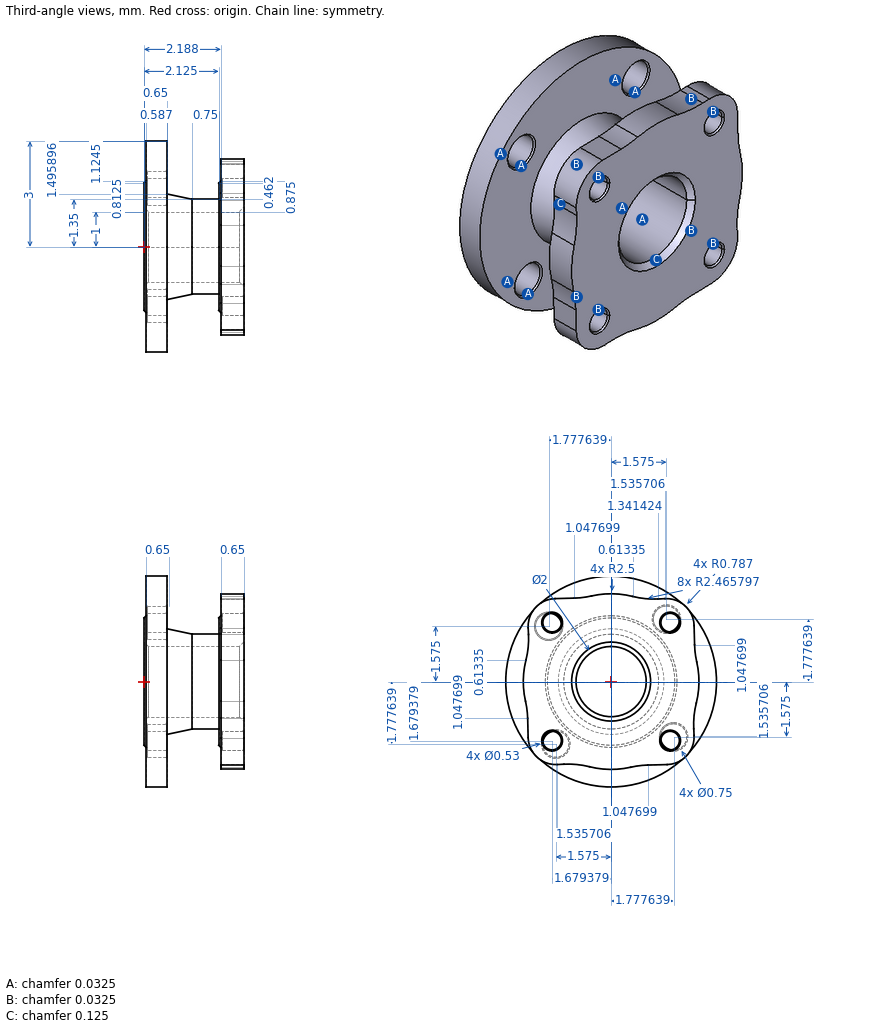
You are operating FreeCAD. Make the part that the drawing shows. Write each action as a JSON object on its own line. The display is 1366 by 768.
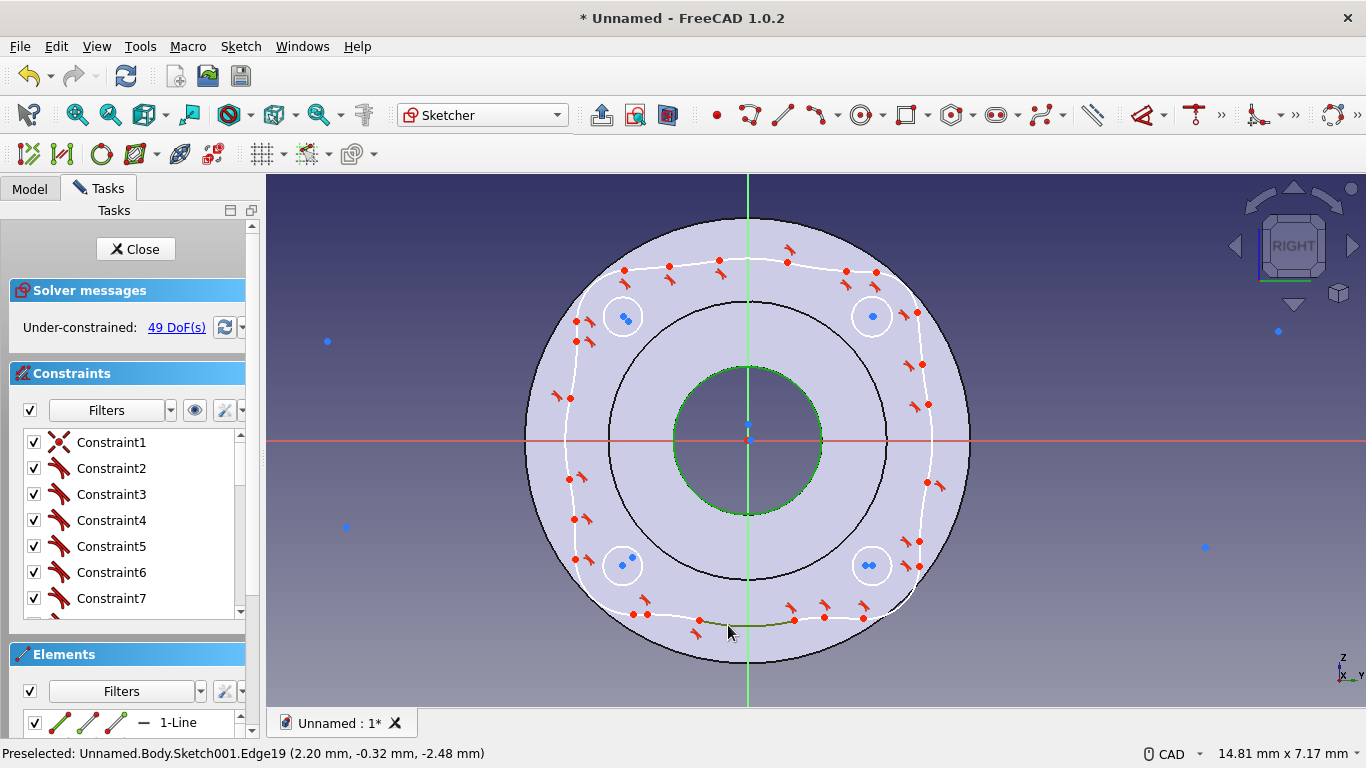
{"action": "left_click", "coordinate": [1194, 116]}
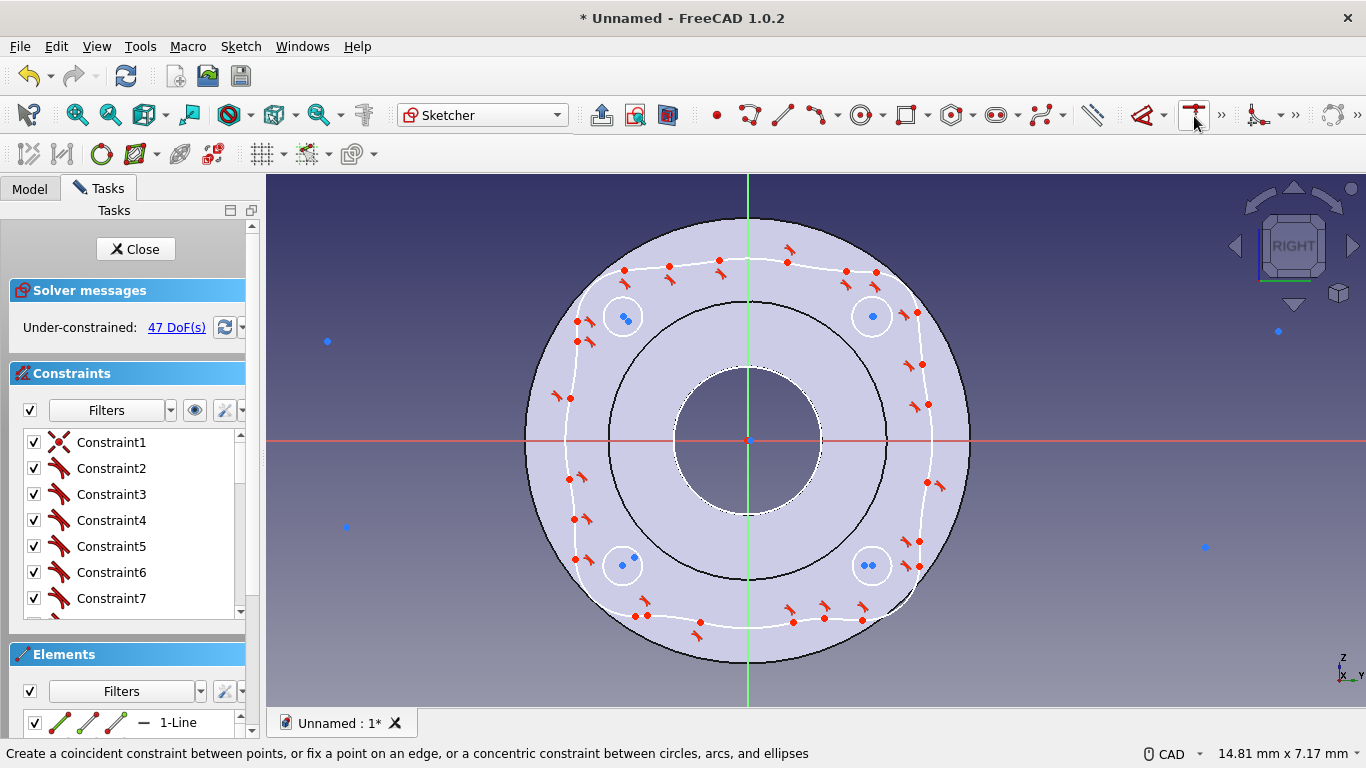
{"action": "left_click", "coordinate": [800, 388]}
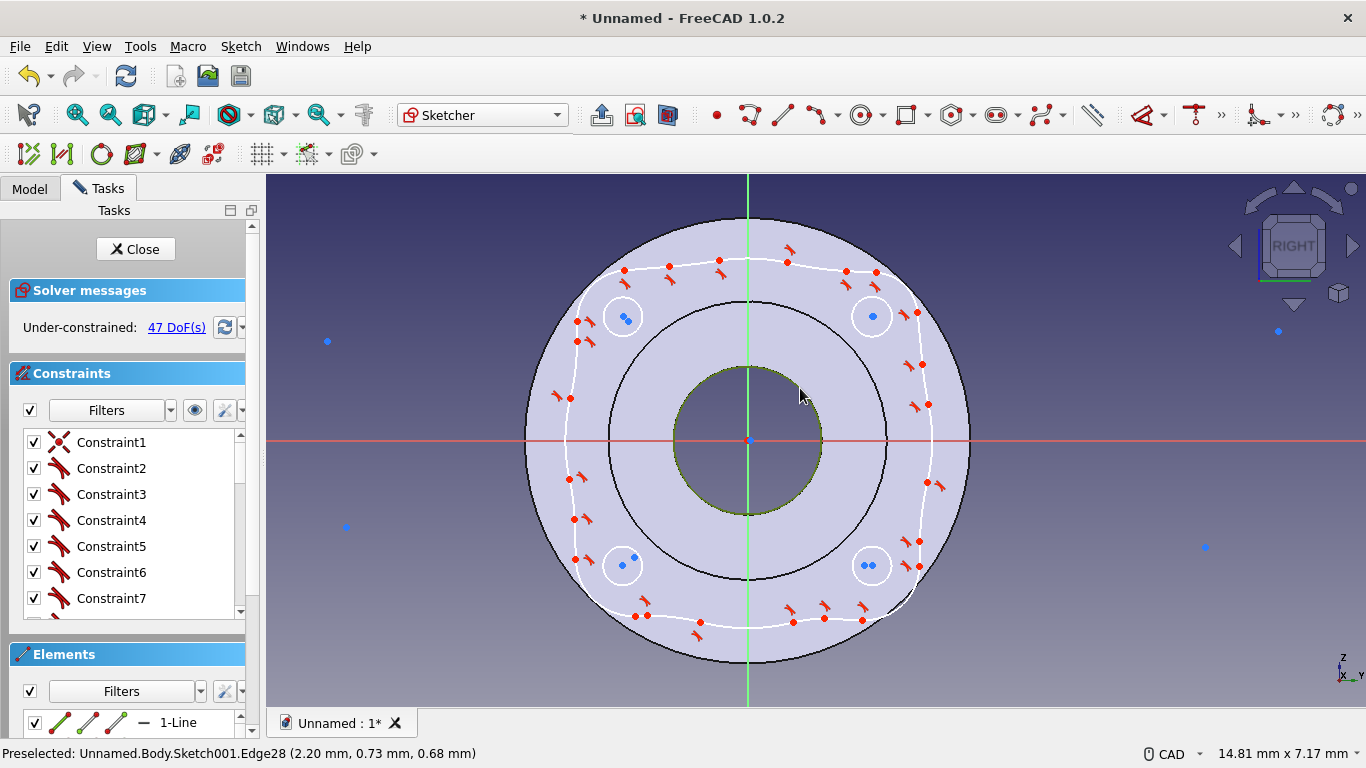
{"action": "left_click", "coordinate": [931, 459]}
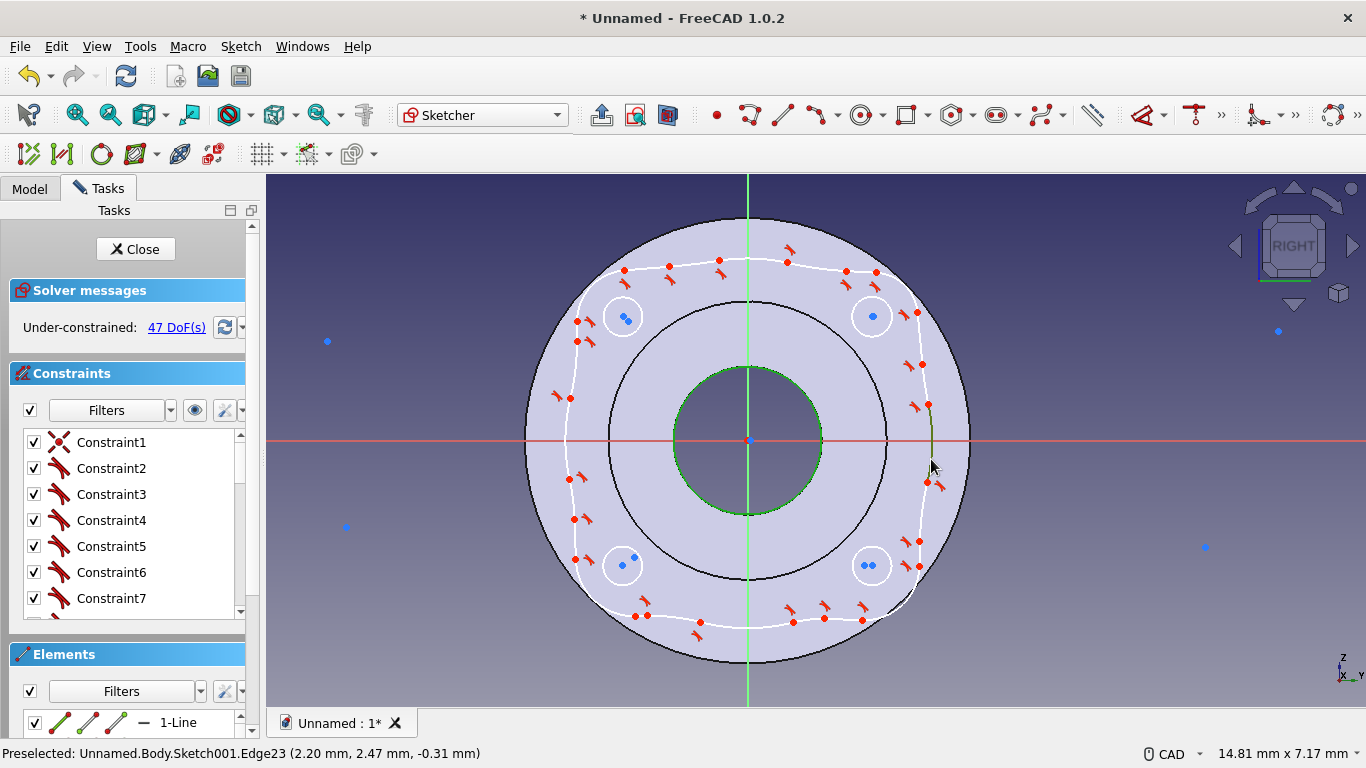
{"action": "left_click", "coordinate": [1194, 116]}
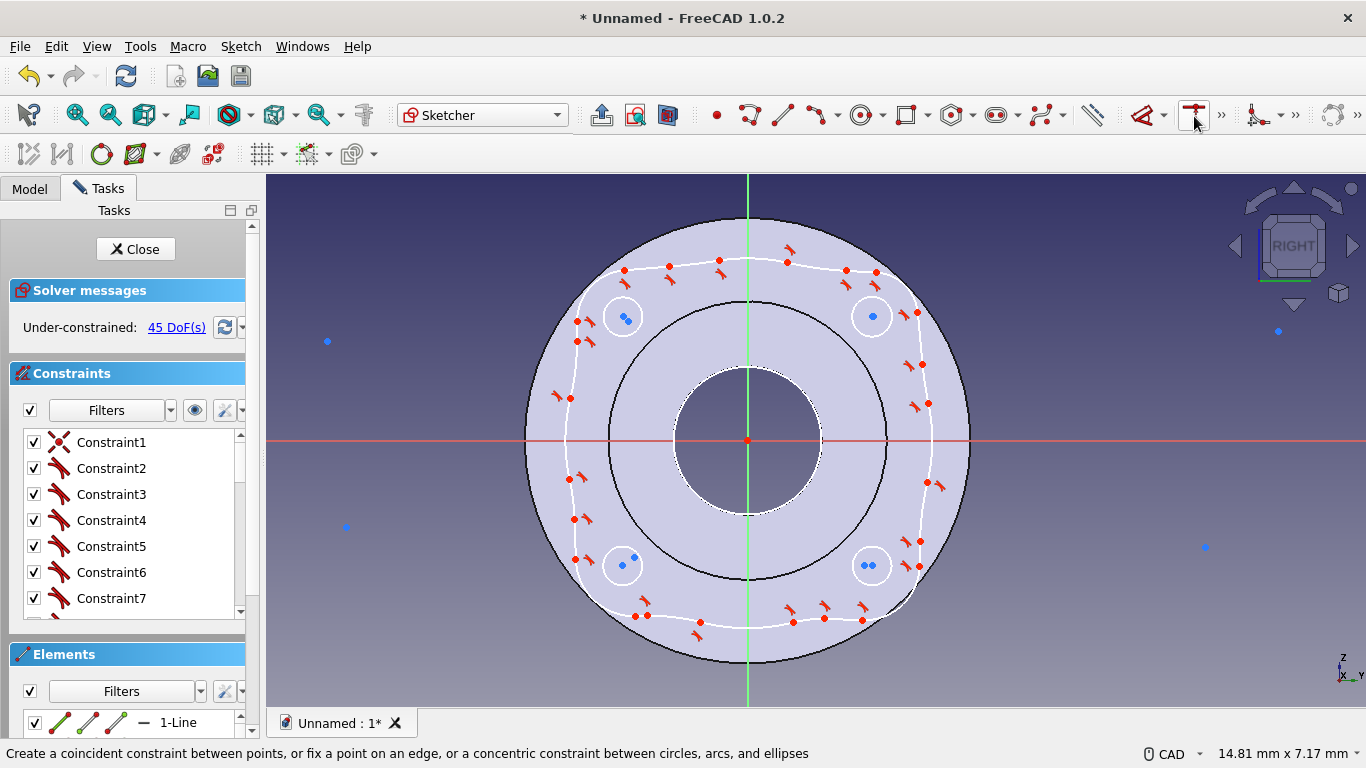
{"action": "left_click", "coordinate": [805, 266]}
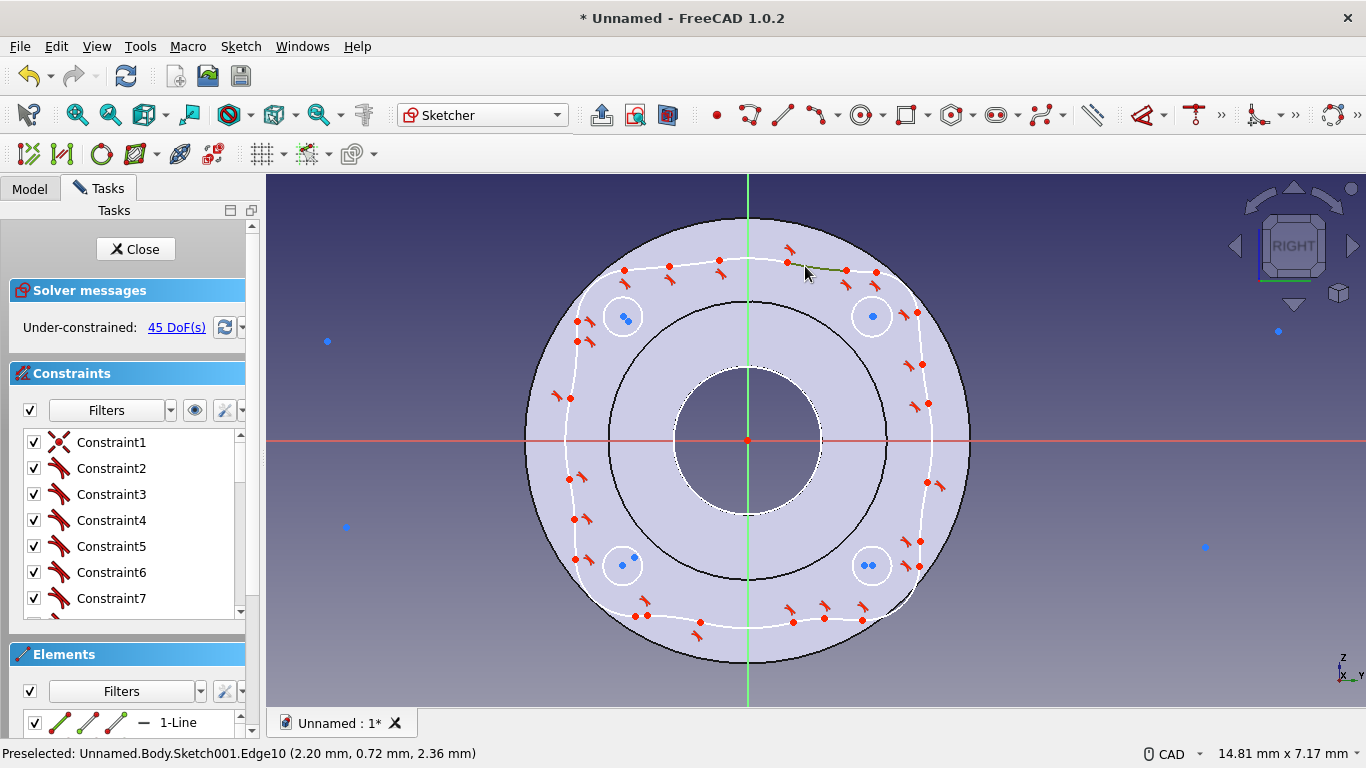
{"action": "left_click", "coordinate": [684, 265]}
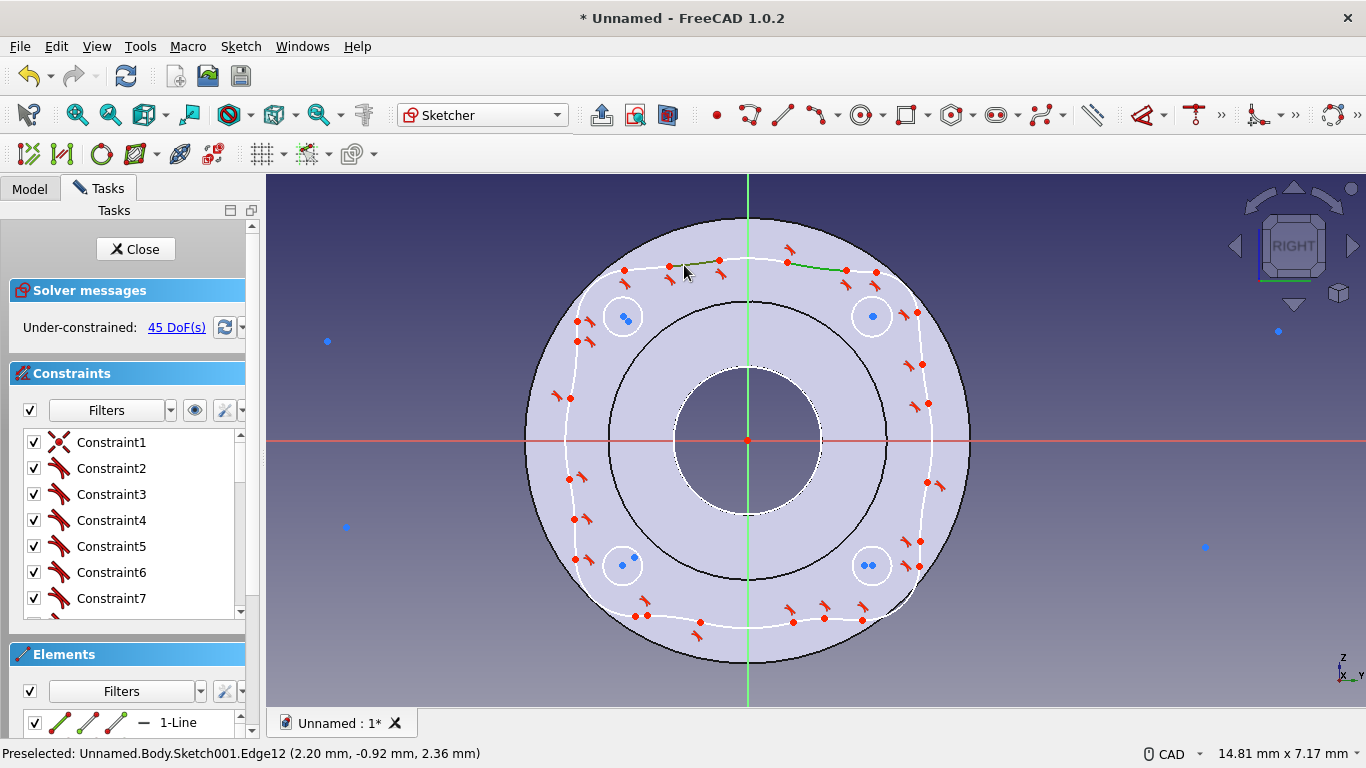
{"action": "left_click", "coordinate": [574, 382]}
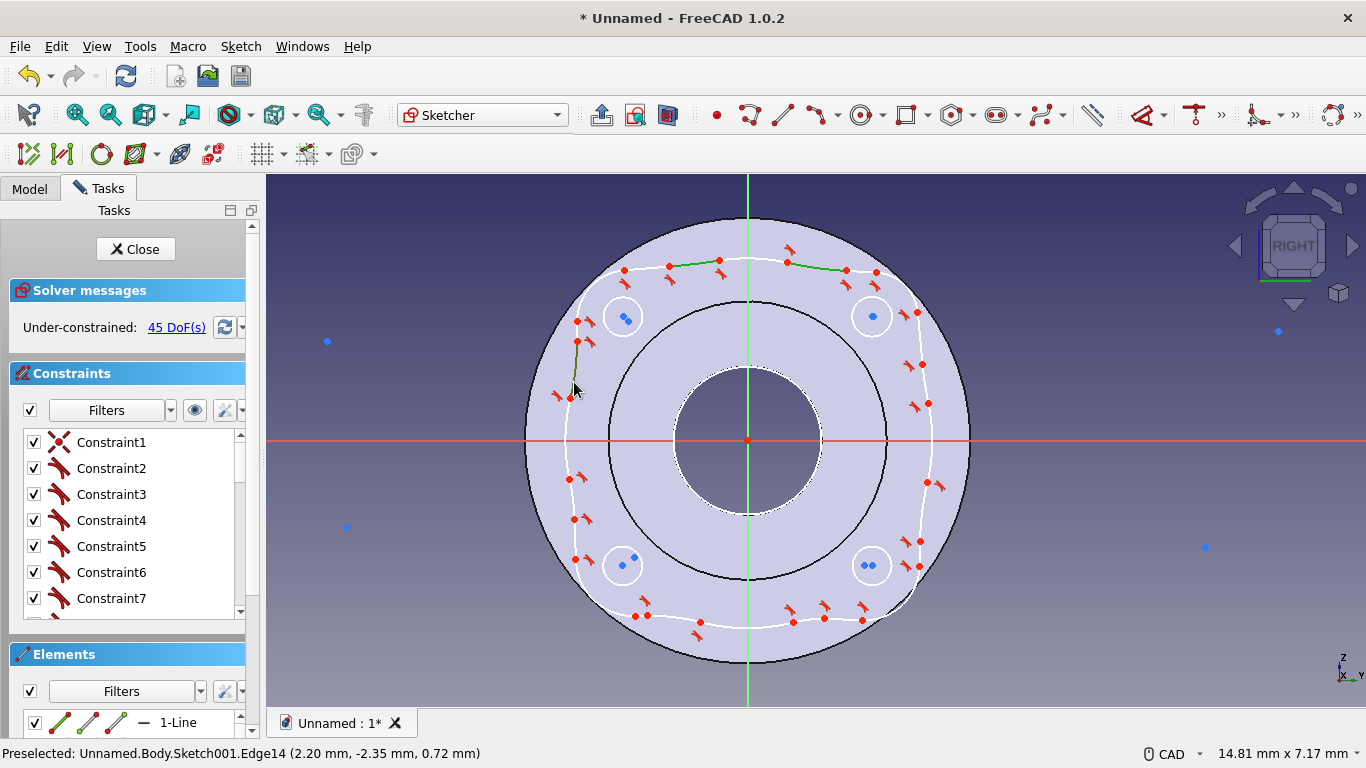
{"action": "left_click", "coordinate": [574, 507]}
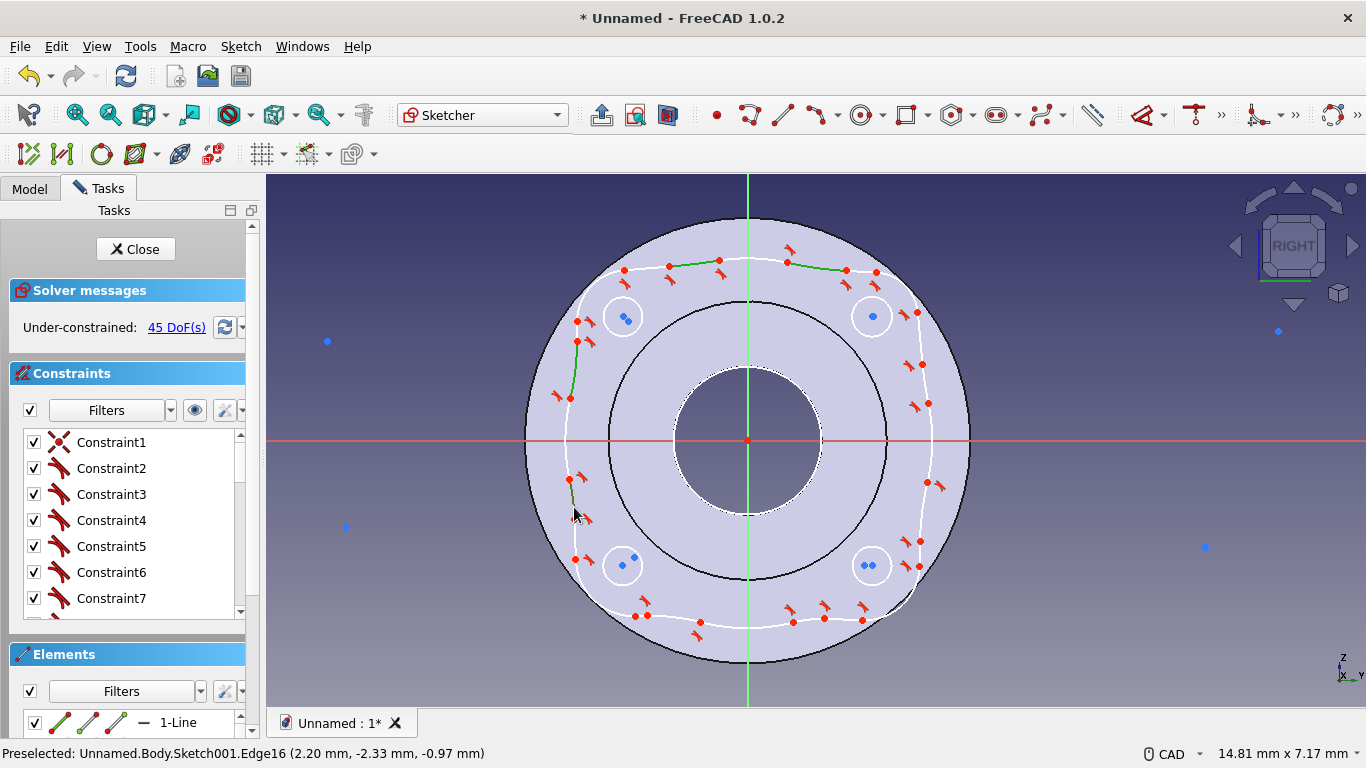
{"action": "left_click", "coordinate": [685, 619]}